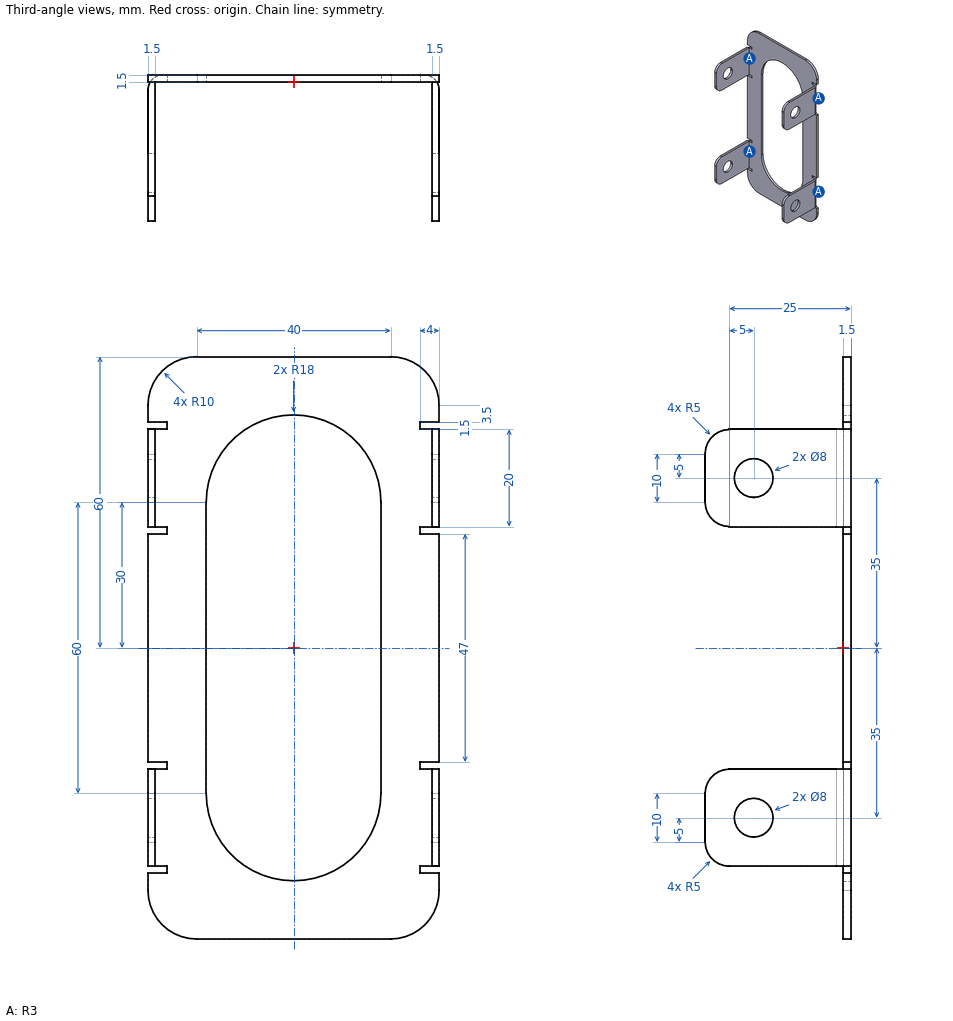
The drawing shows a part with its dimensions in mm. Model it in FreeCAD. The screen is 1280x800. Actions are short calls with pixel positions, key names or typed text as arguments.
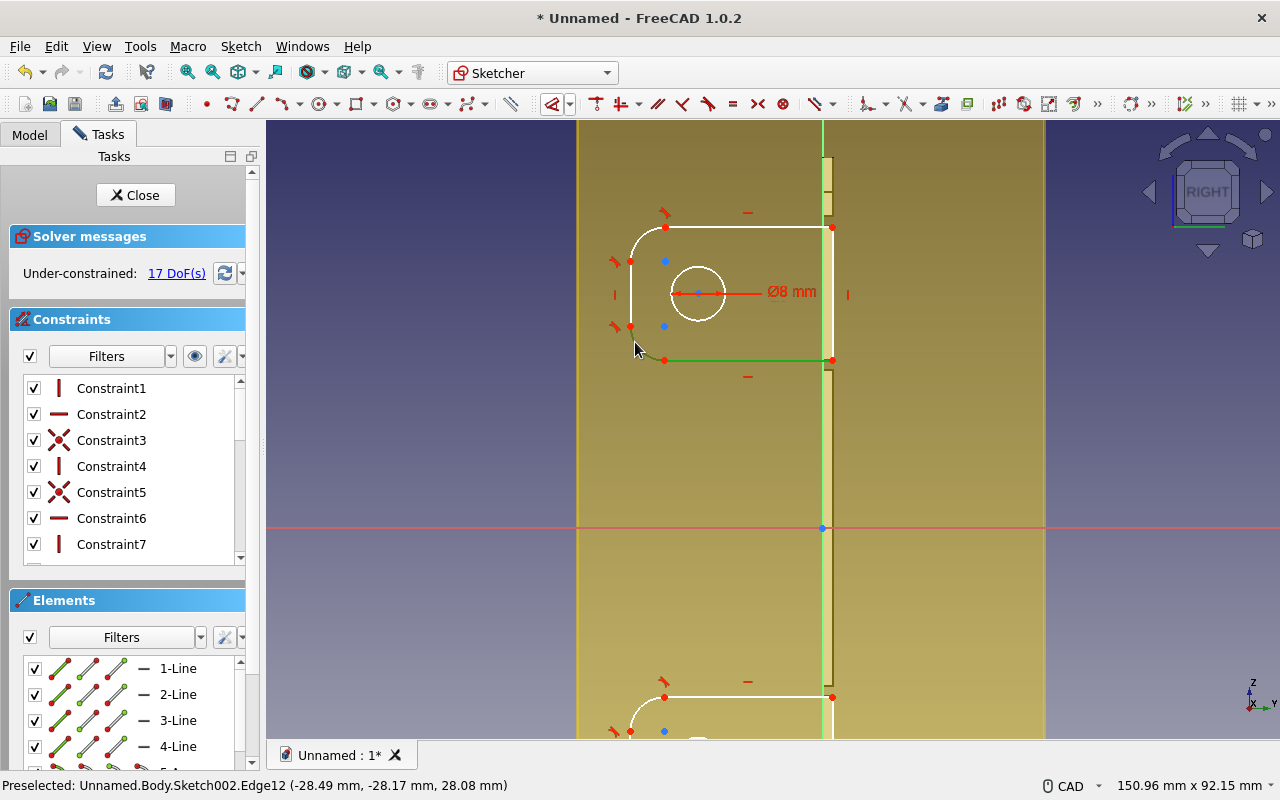
click(708, 104)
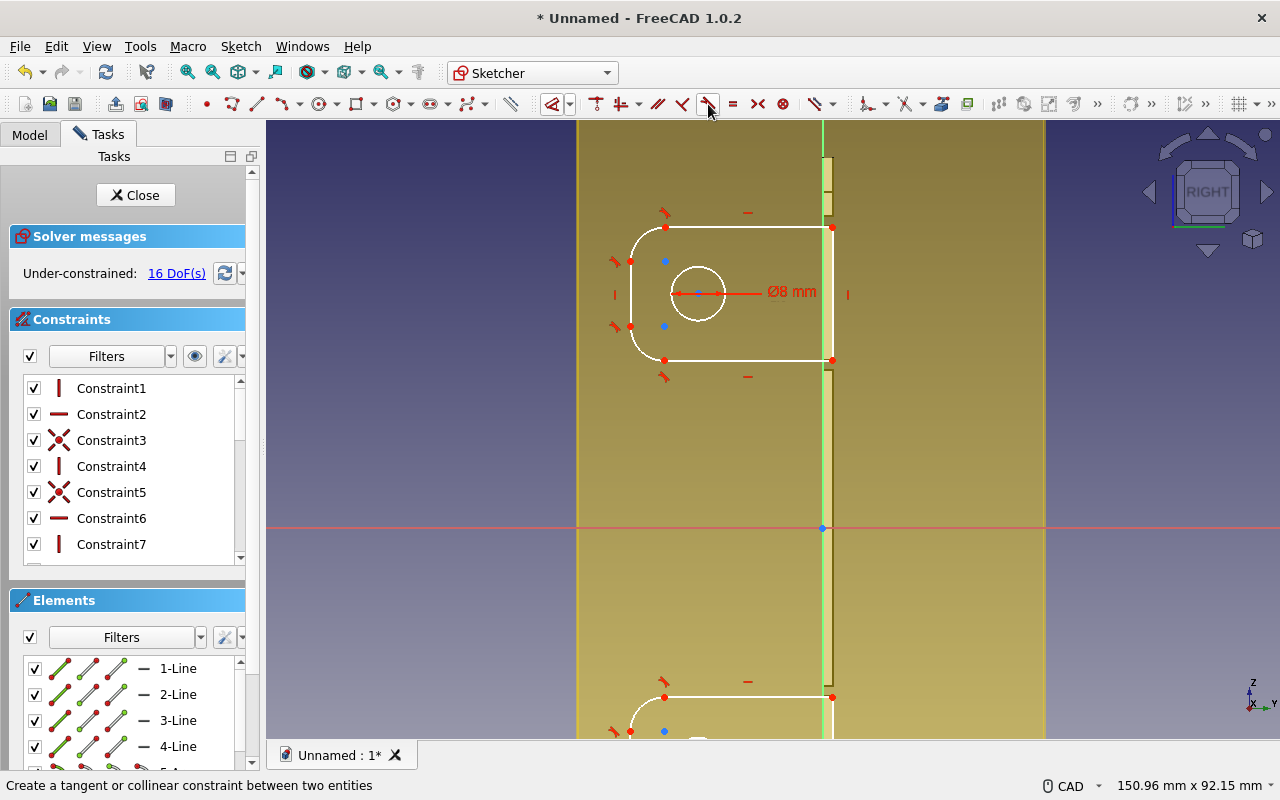
click(649, 701)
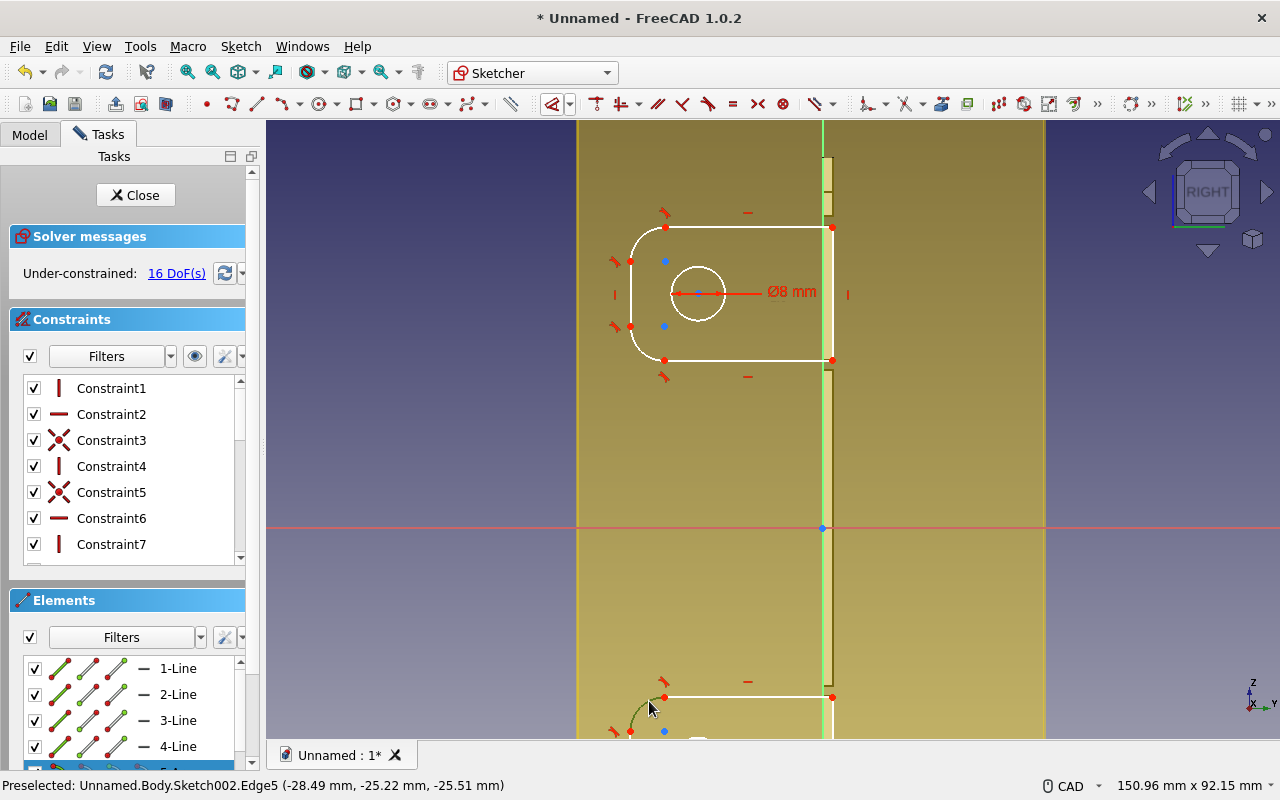
scroll(649, 229, down, 2)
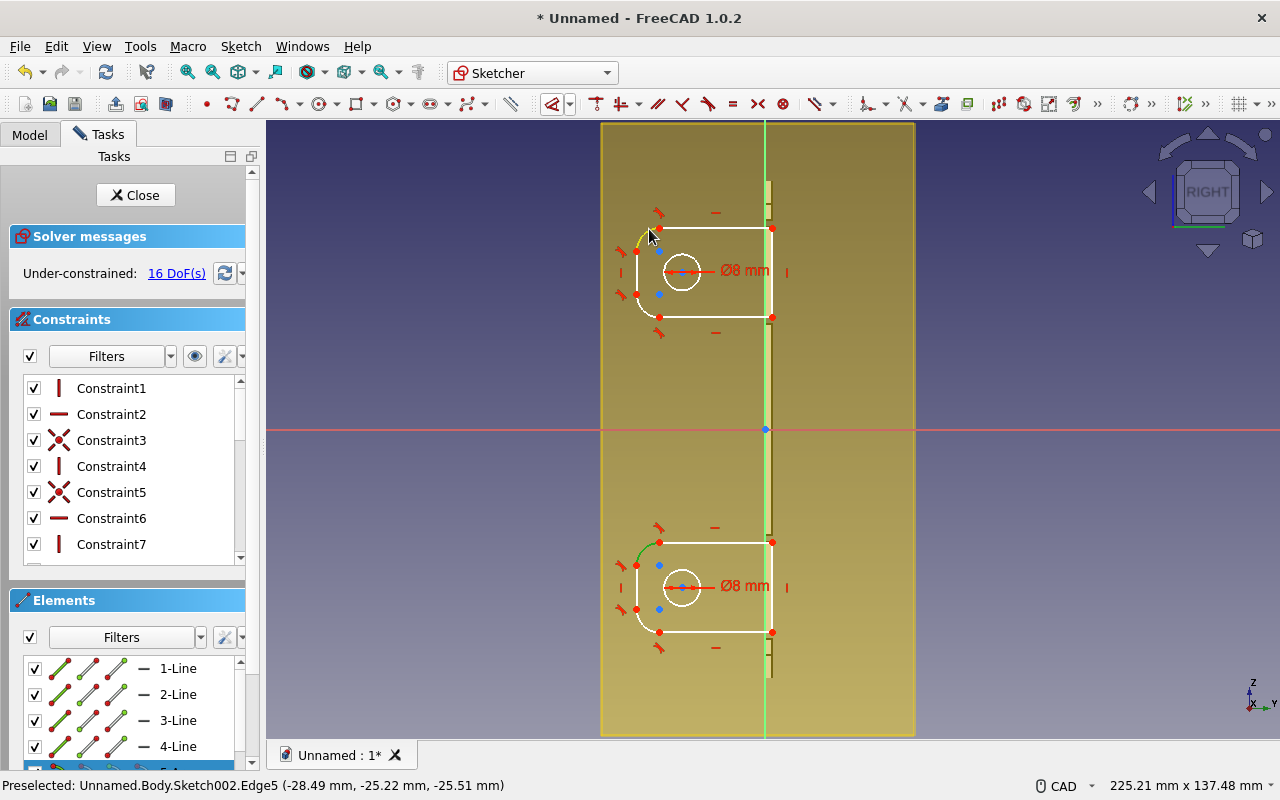
scroll(639, 620, up, 2)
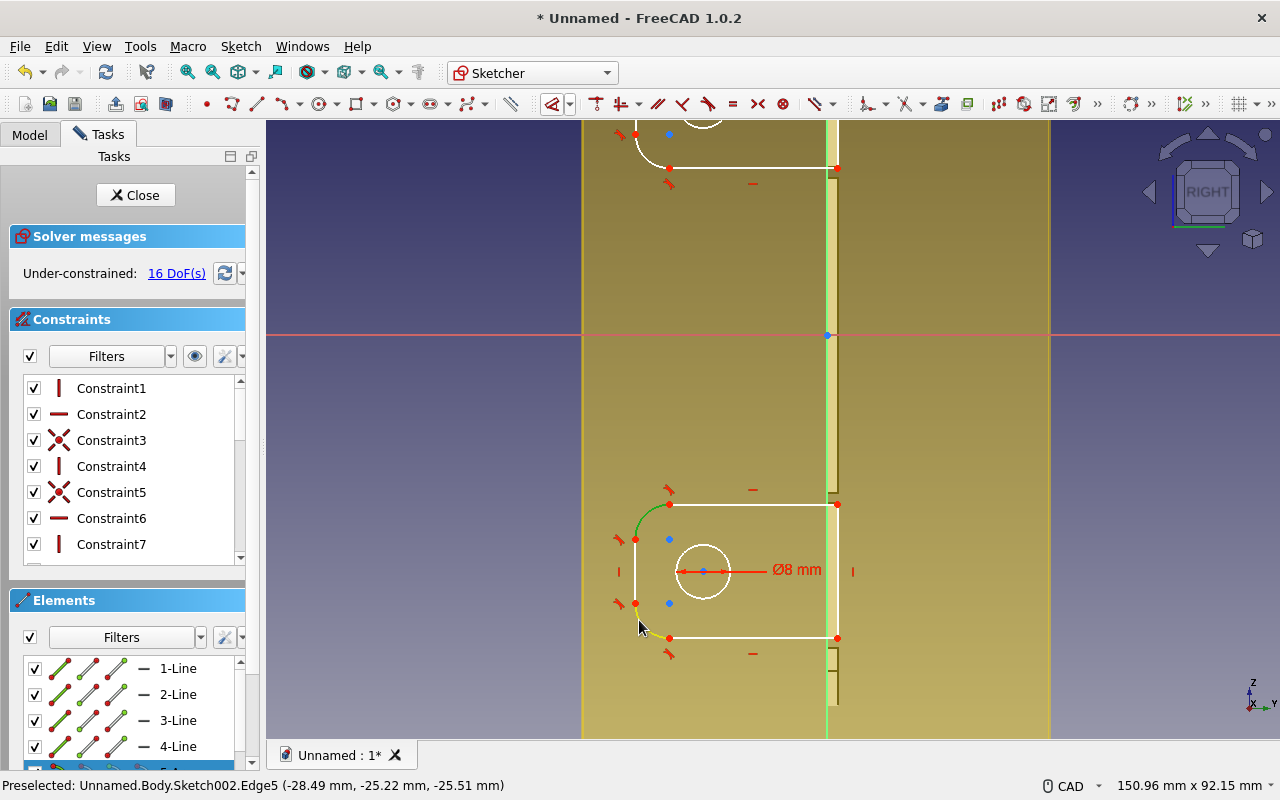
click(639, 619)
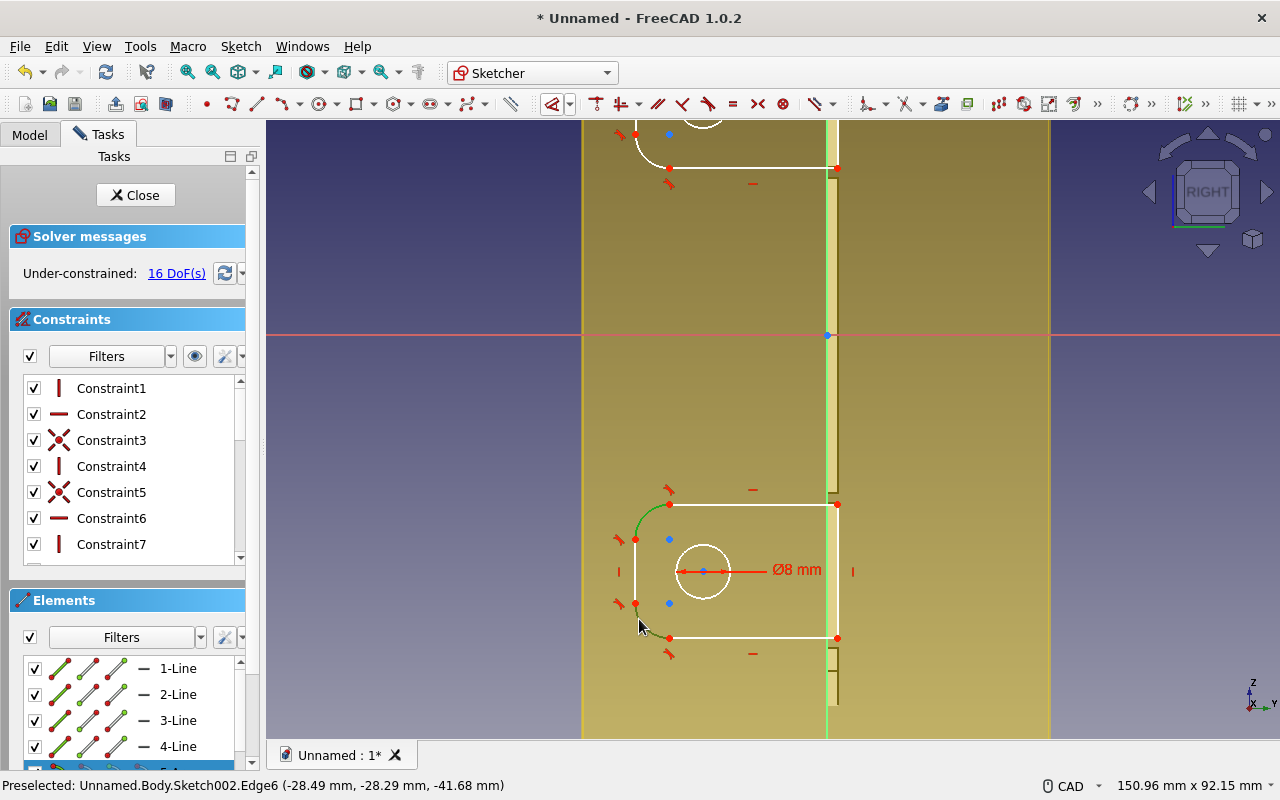
scroll(639, 621, down, 2)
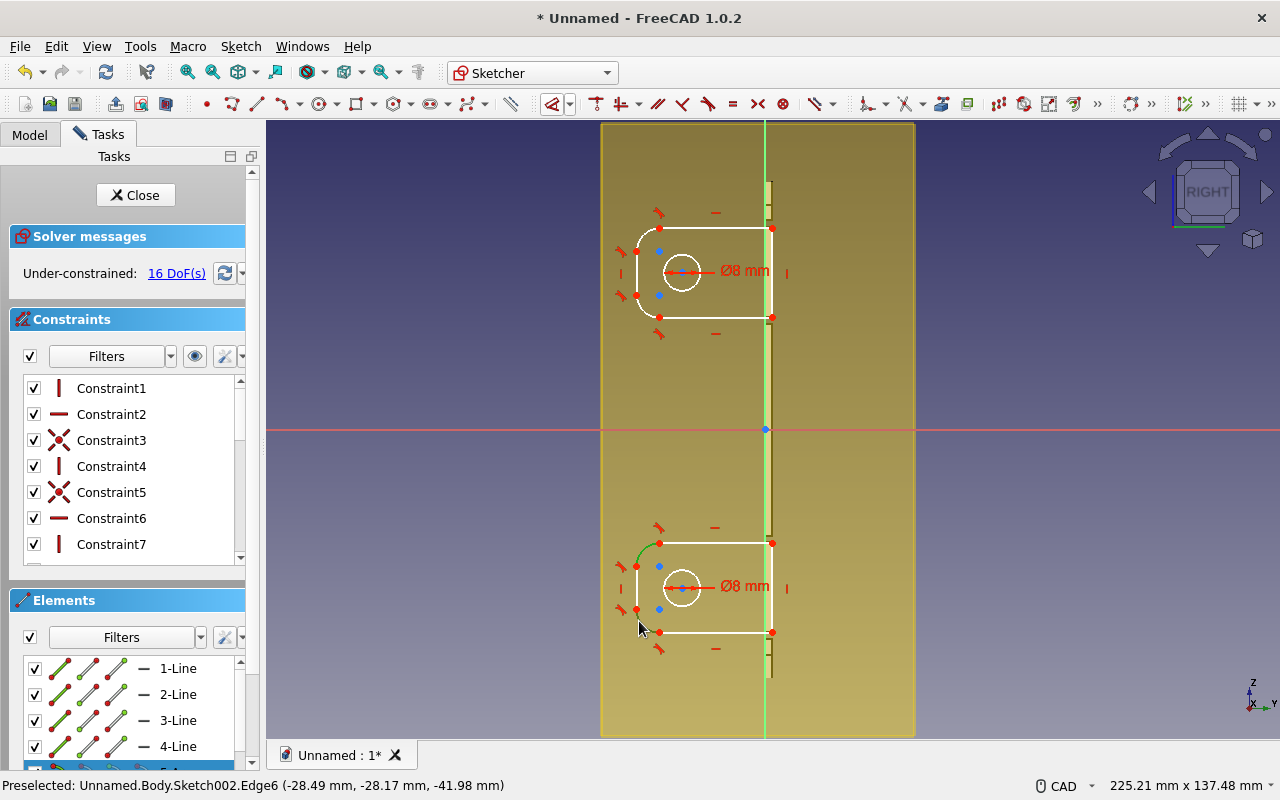
scroll(650, 231, up, 2)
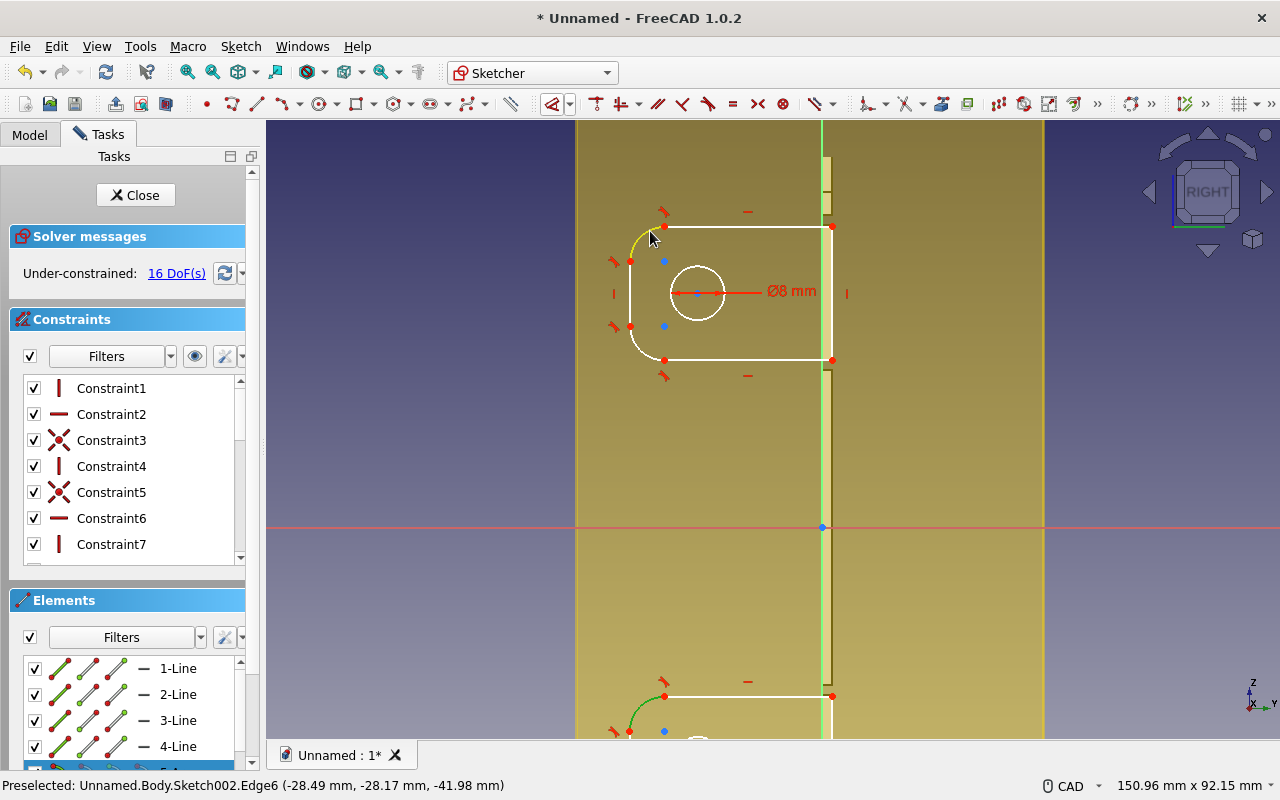
click(649, 231)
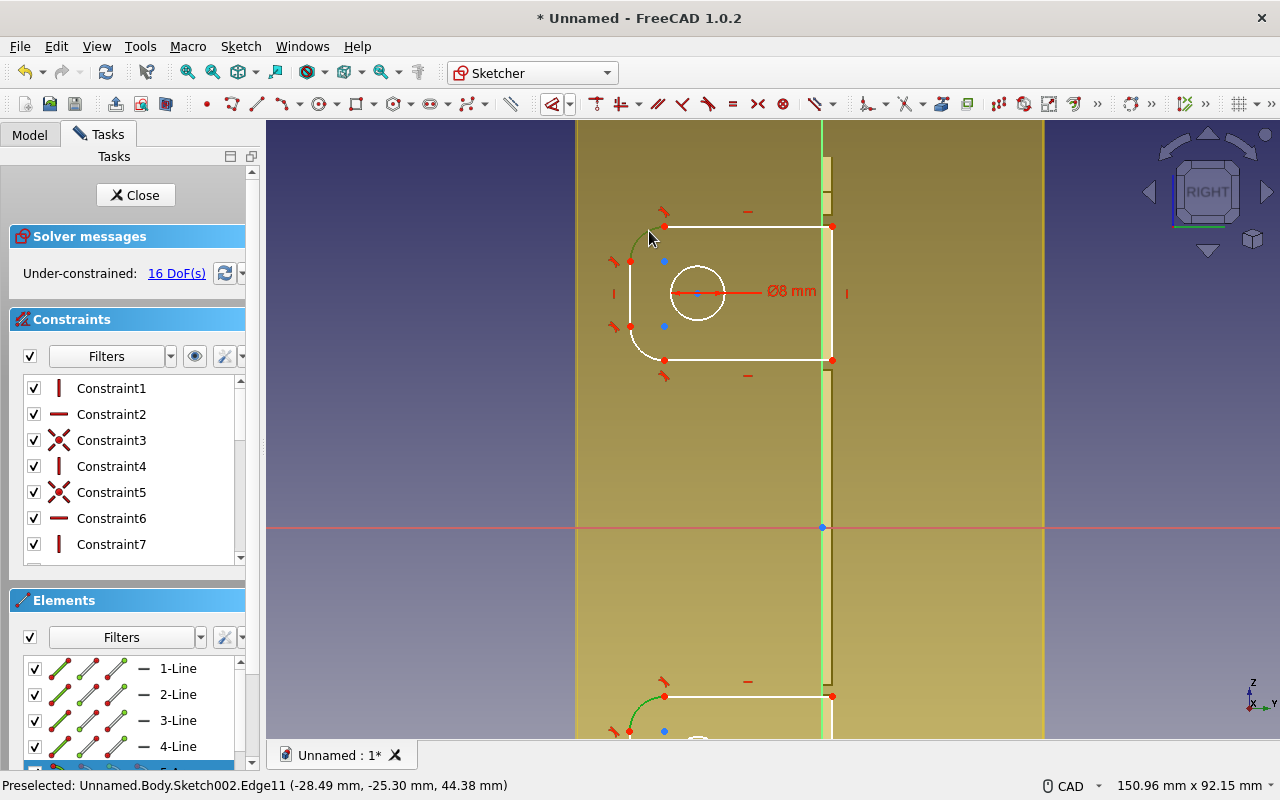
click(634, 342)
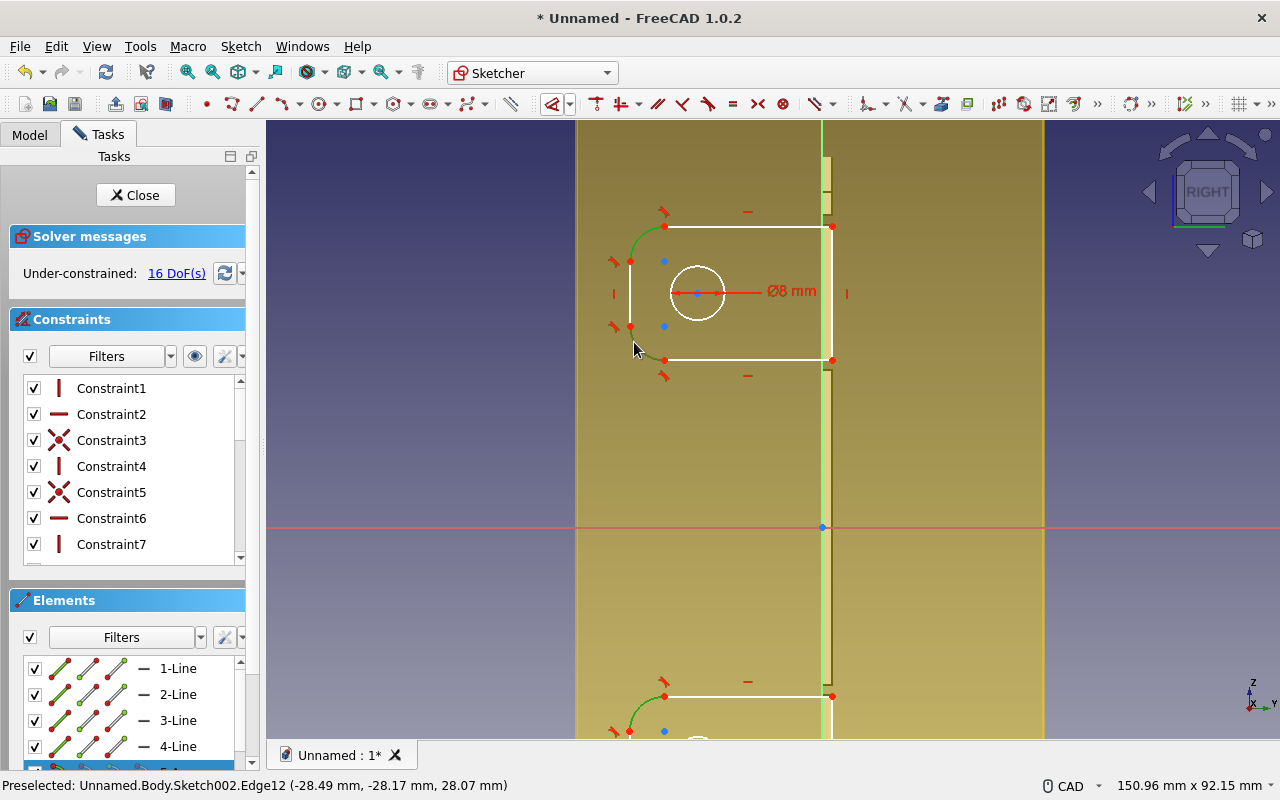
click(733, 104)